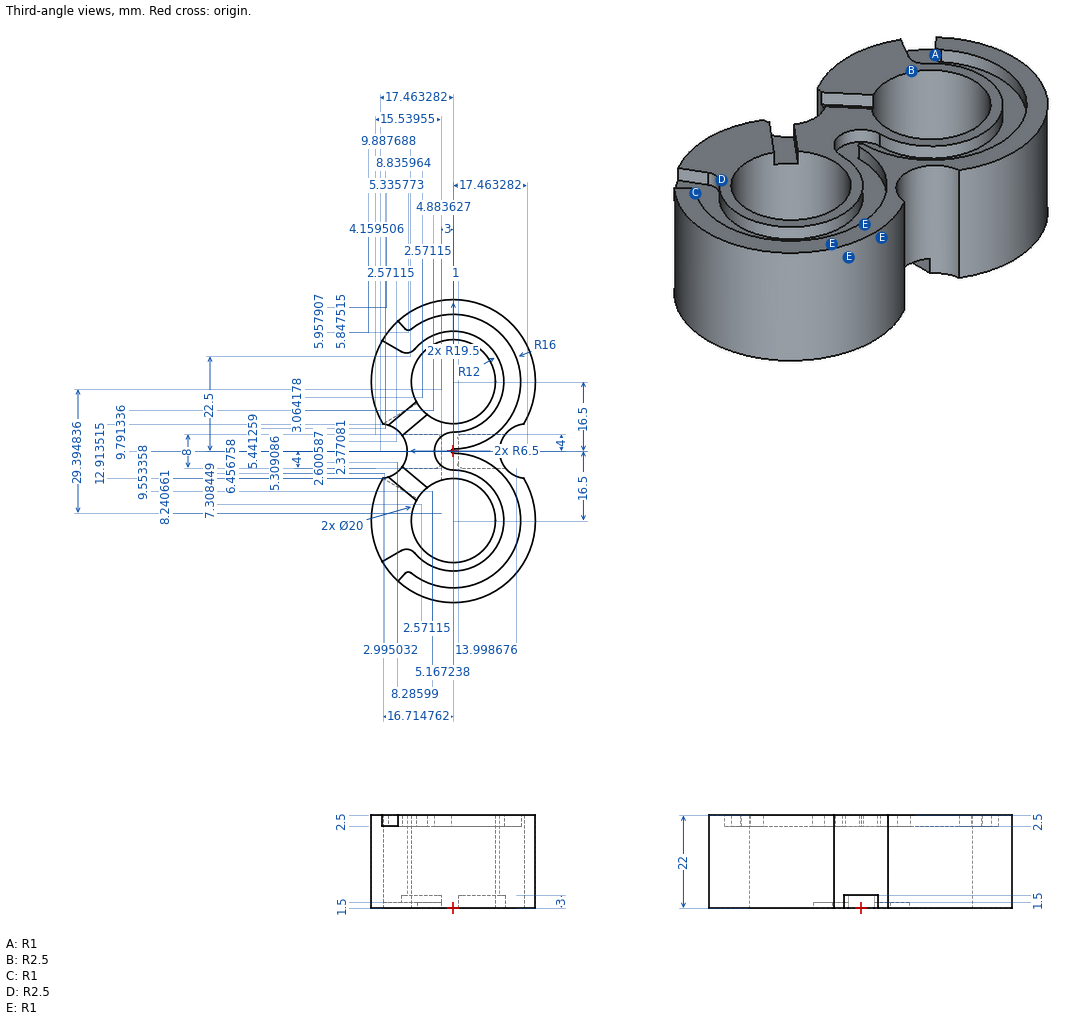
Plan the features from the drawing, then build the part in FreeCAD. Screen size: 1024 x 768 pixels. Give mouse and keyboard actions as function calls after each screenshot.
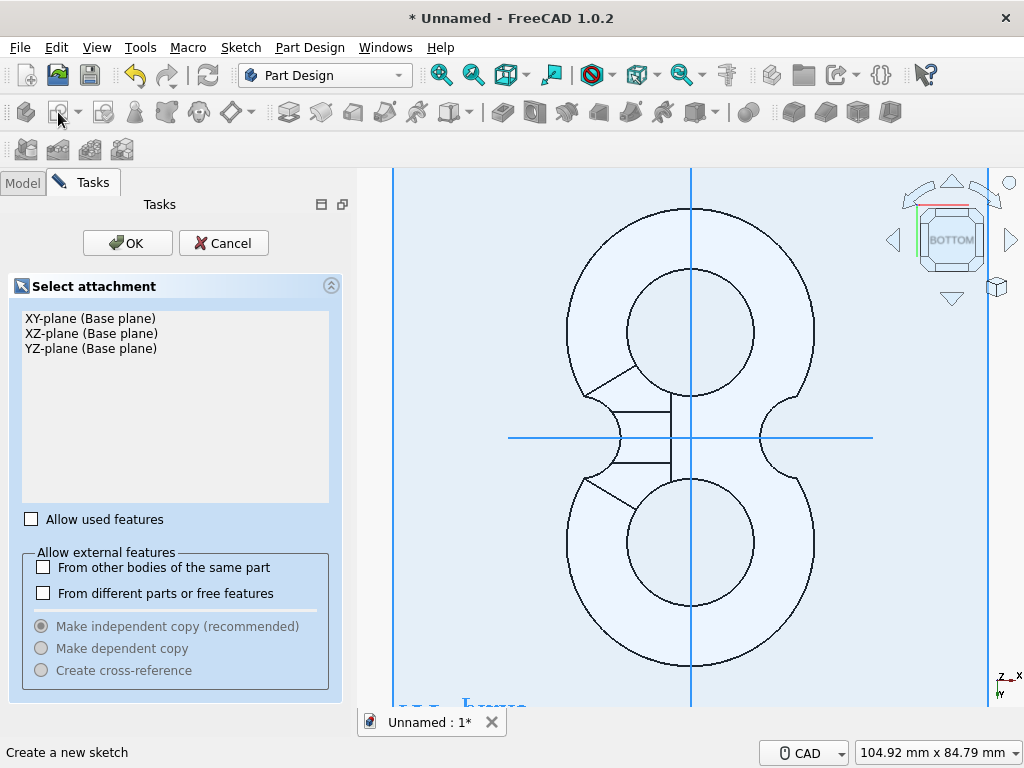
click(82, 318)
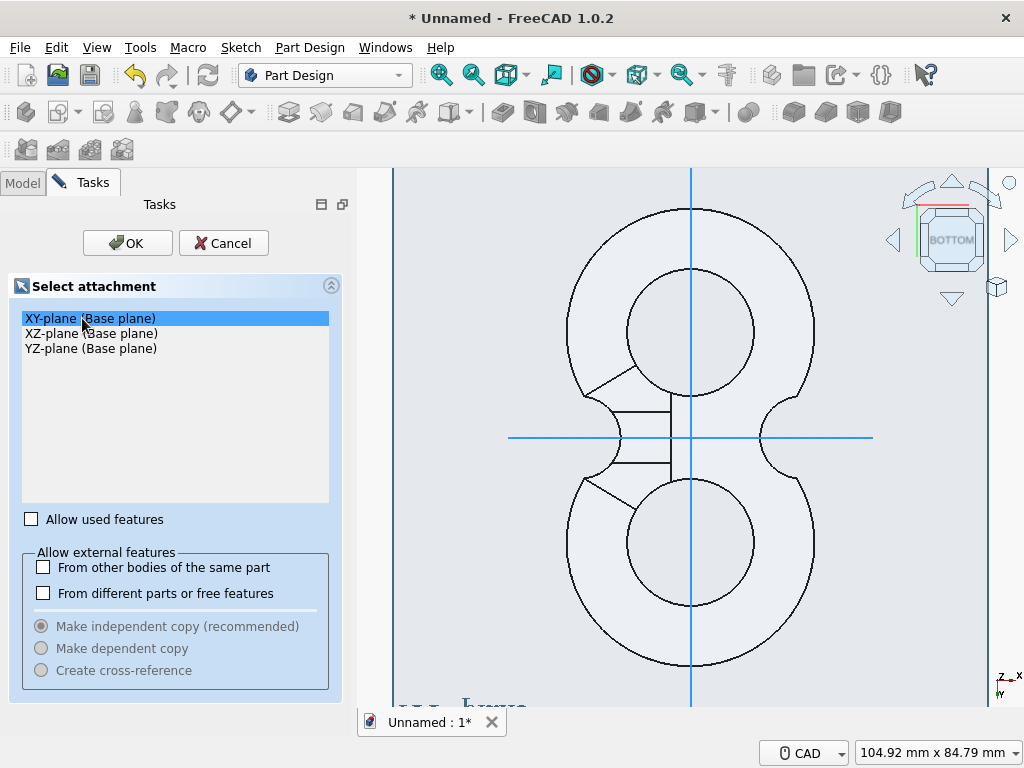
click(128, 243)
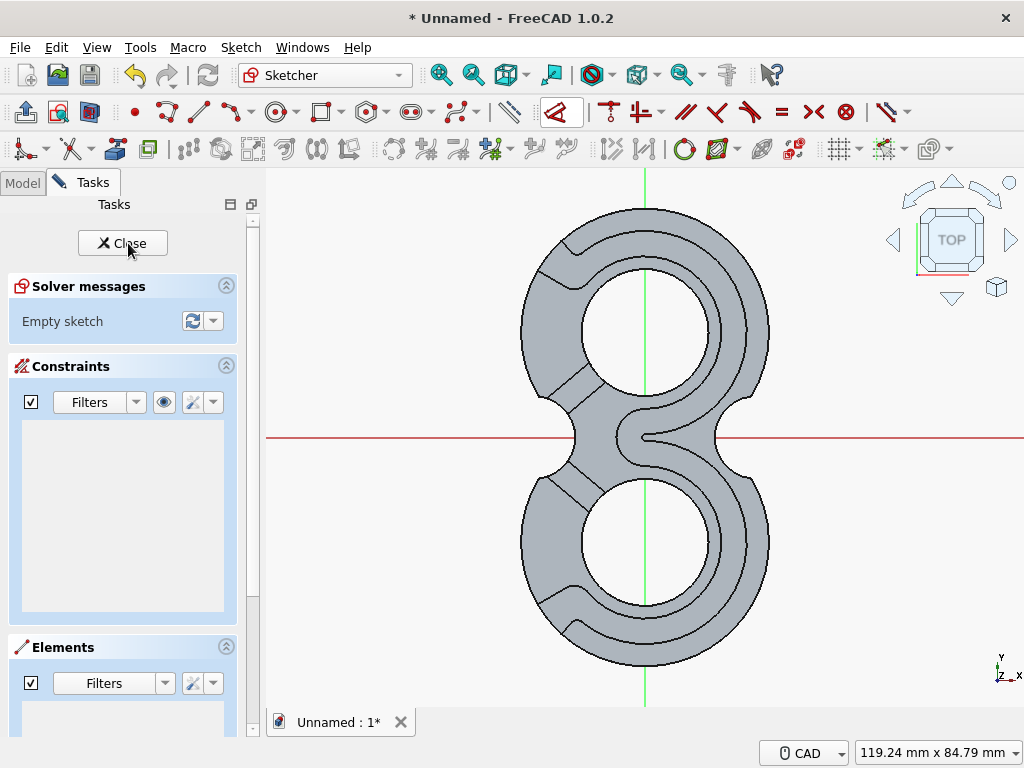
key(q)
key(s)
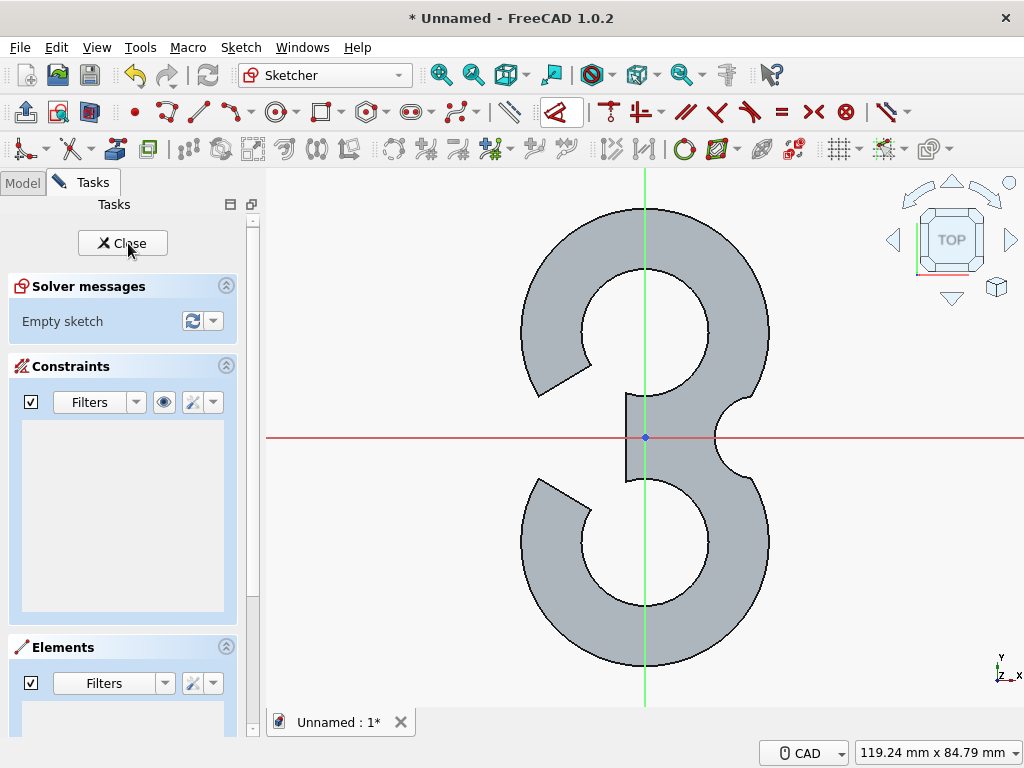
scroll(731, 437, up, 7)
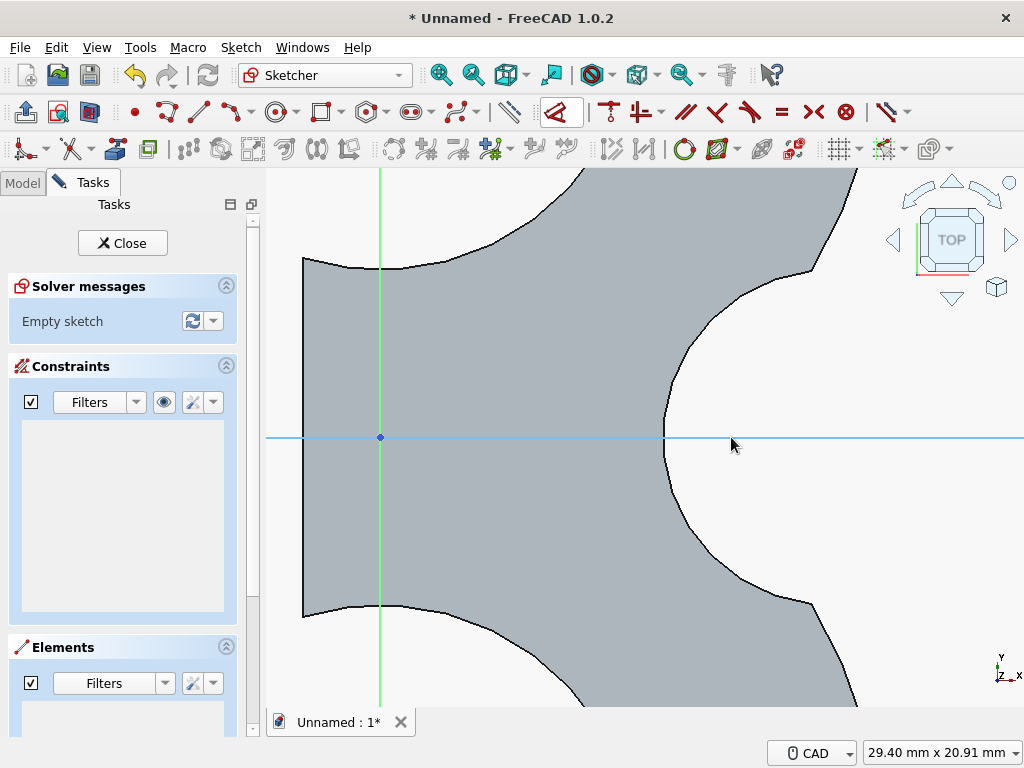
click(322, 112)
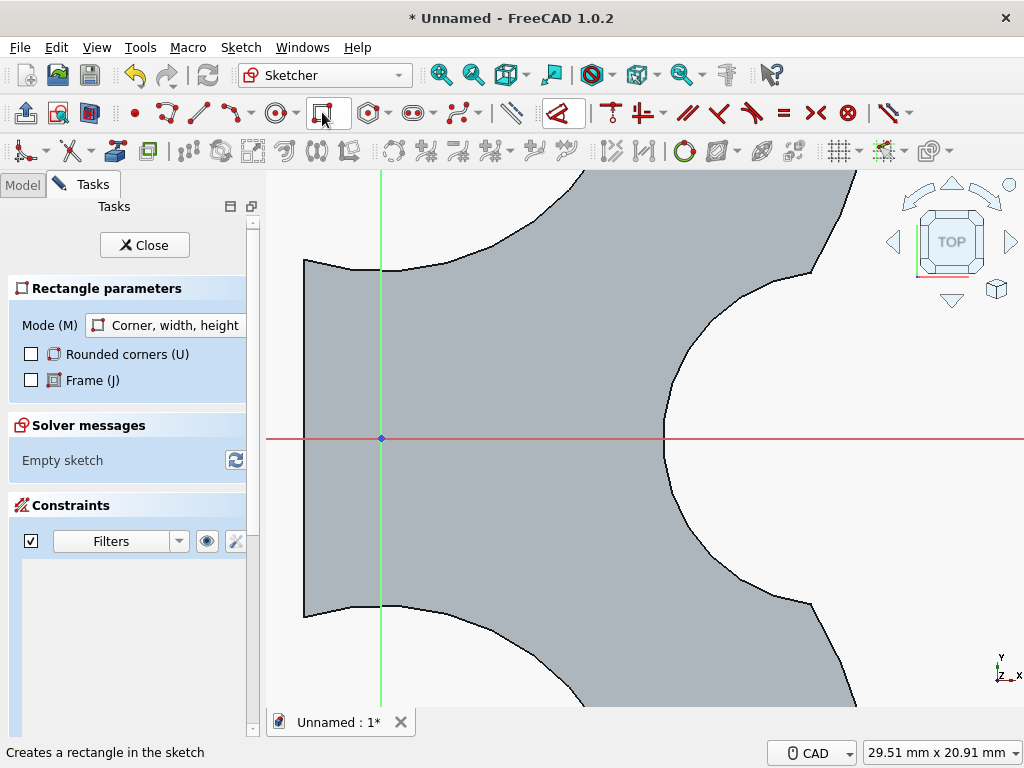
click(407, 336)
move(767, 541)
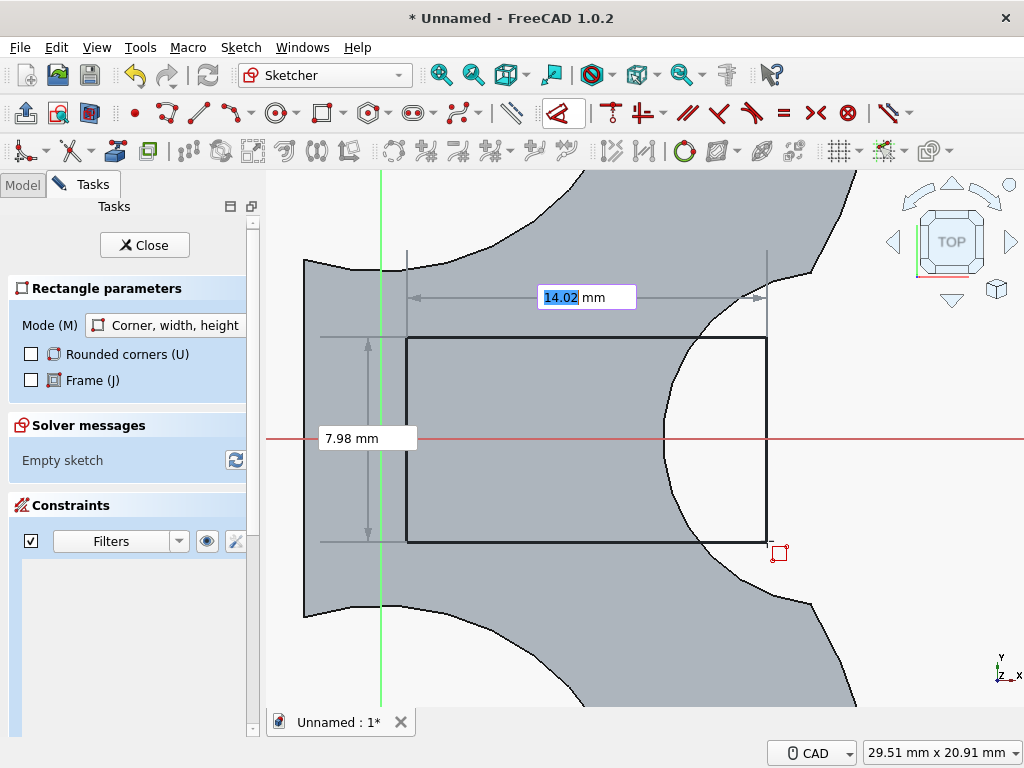
text(13.998676)
key(Tab)
text(8)
key(Return)
key(Escape)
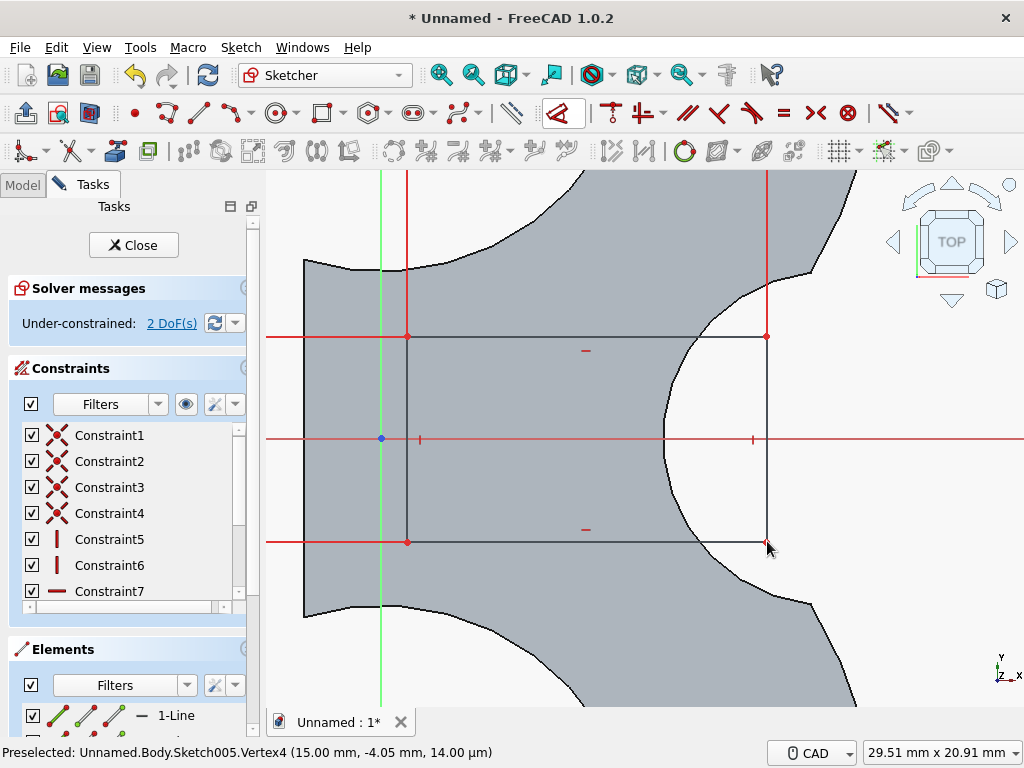
scroll(407, 337, up, 3)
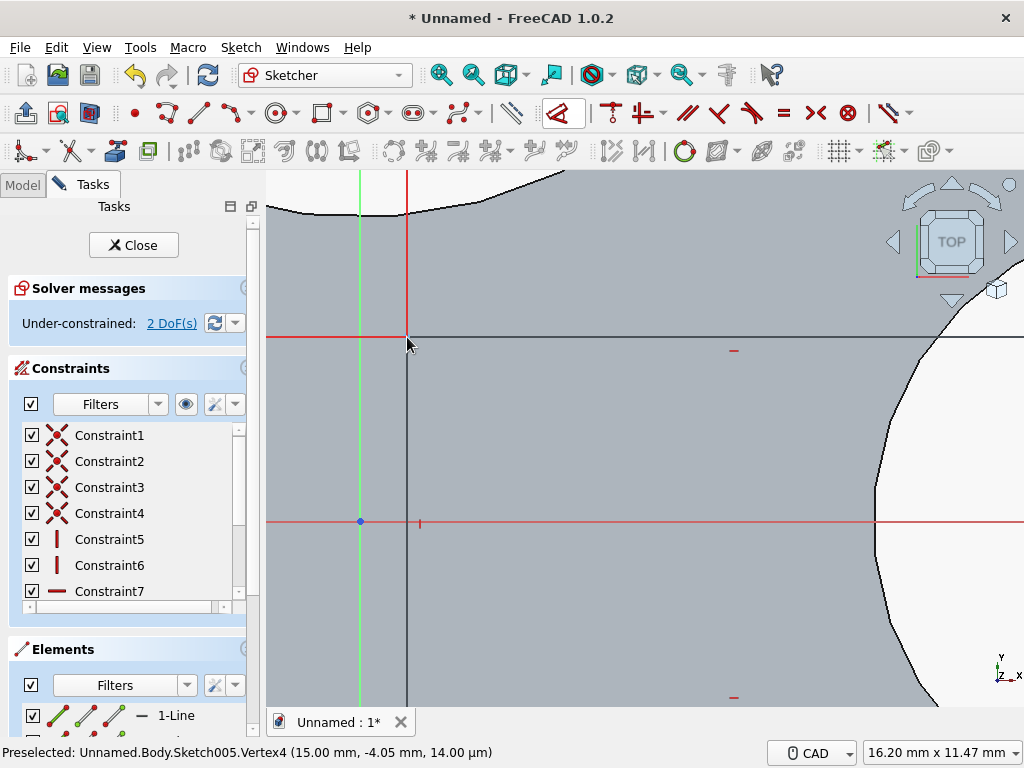
click(407, 337)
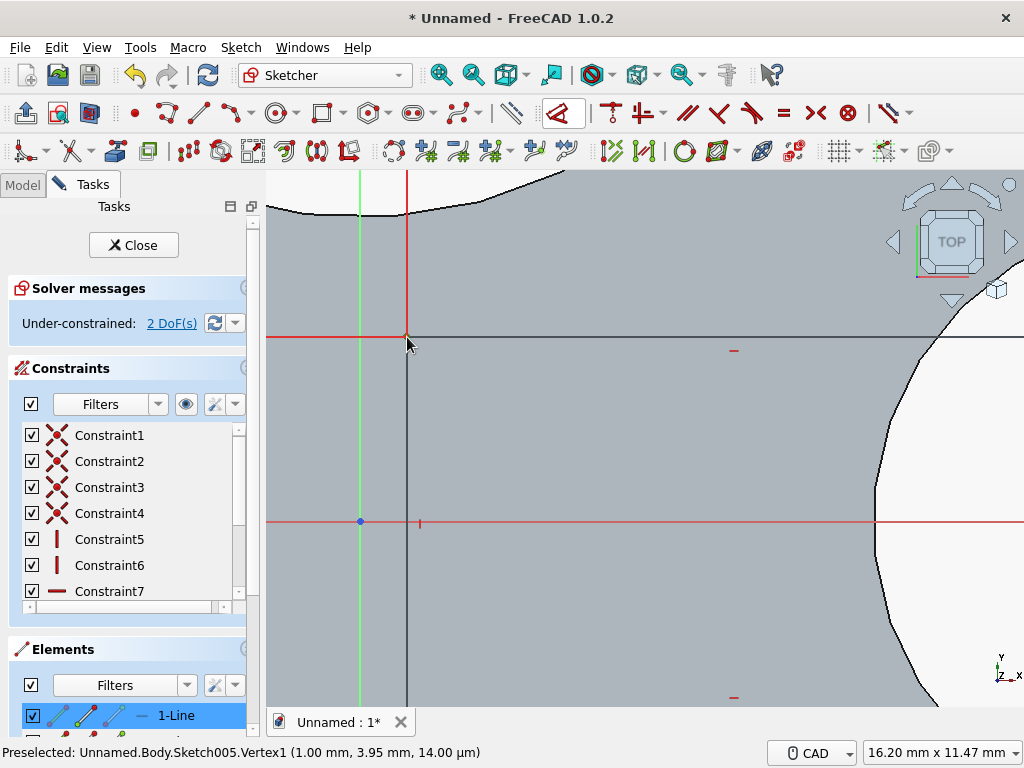
key(l)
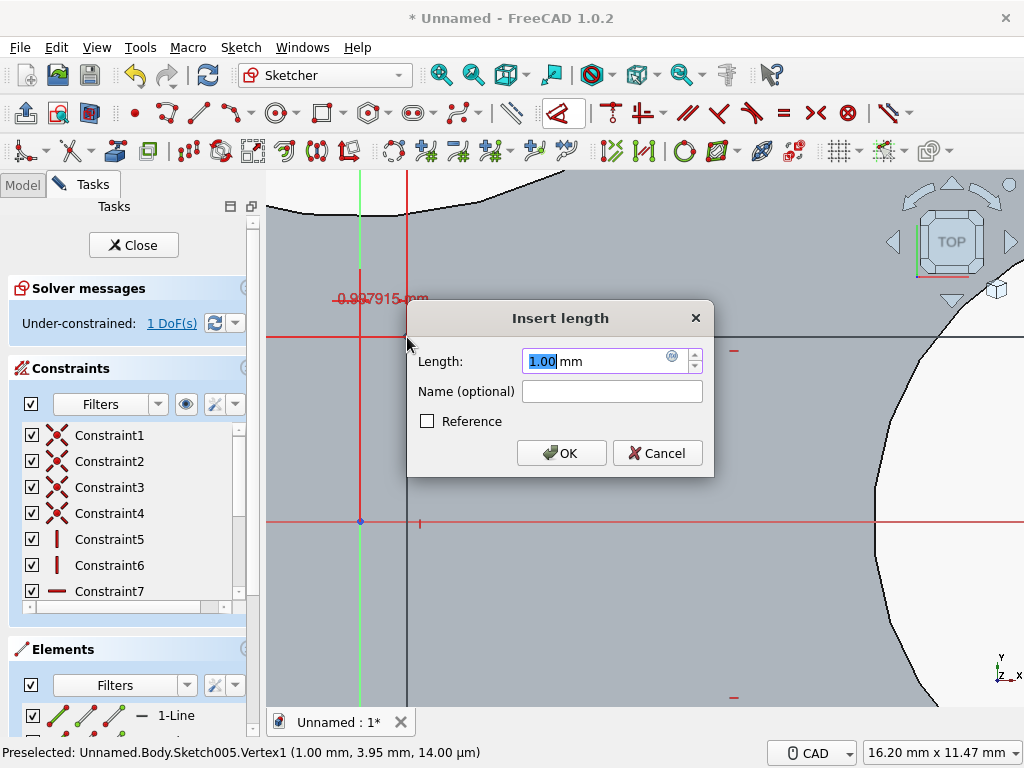
text(1)
key(Return)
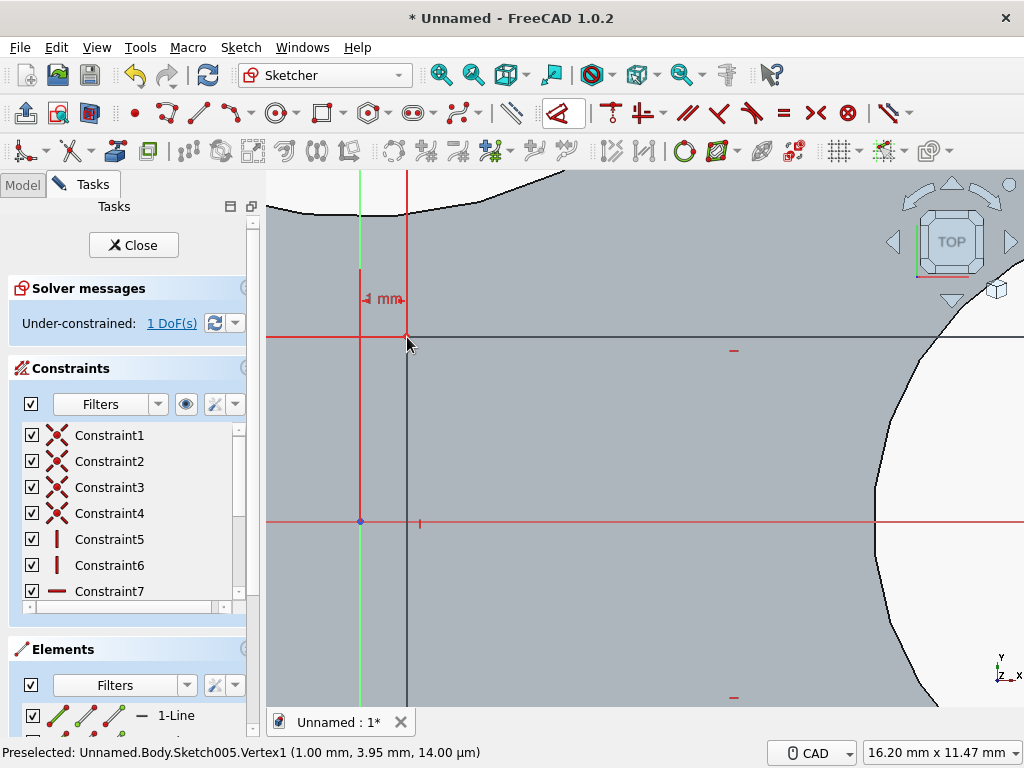
click(407, 337)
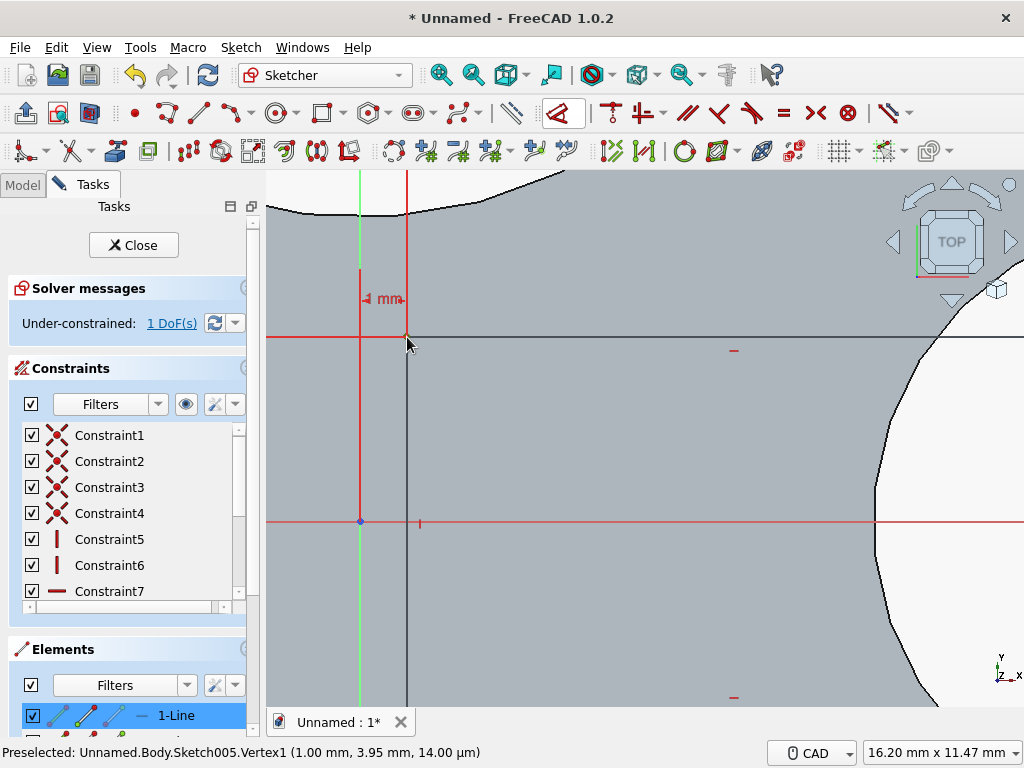
click(580, 114)